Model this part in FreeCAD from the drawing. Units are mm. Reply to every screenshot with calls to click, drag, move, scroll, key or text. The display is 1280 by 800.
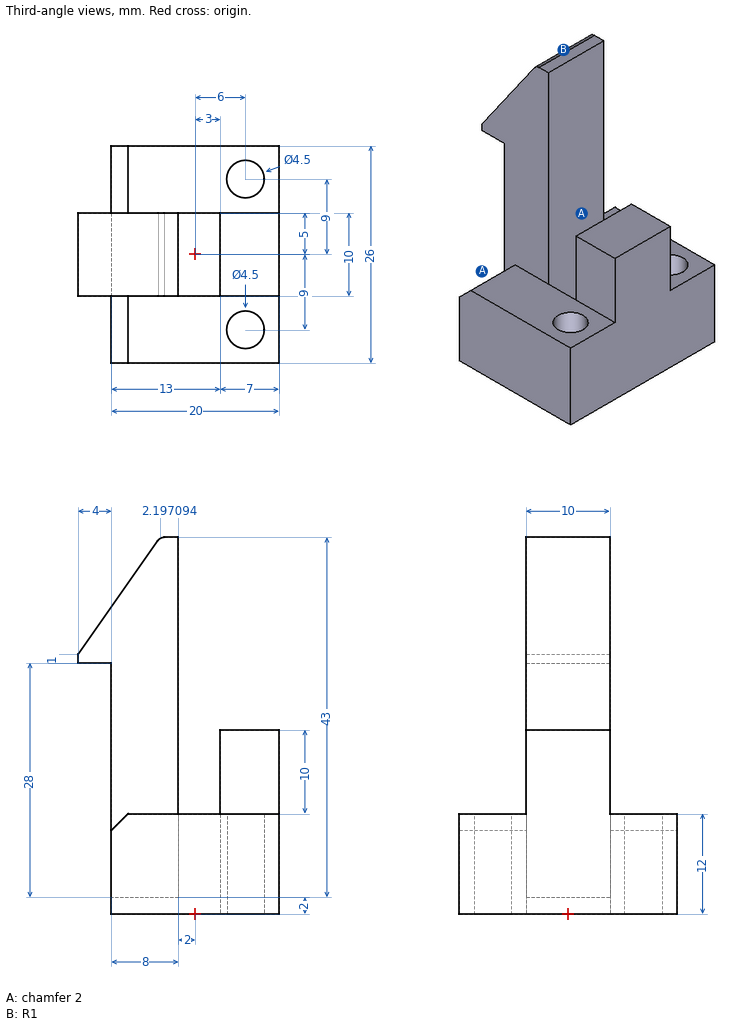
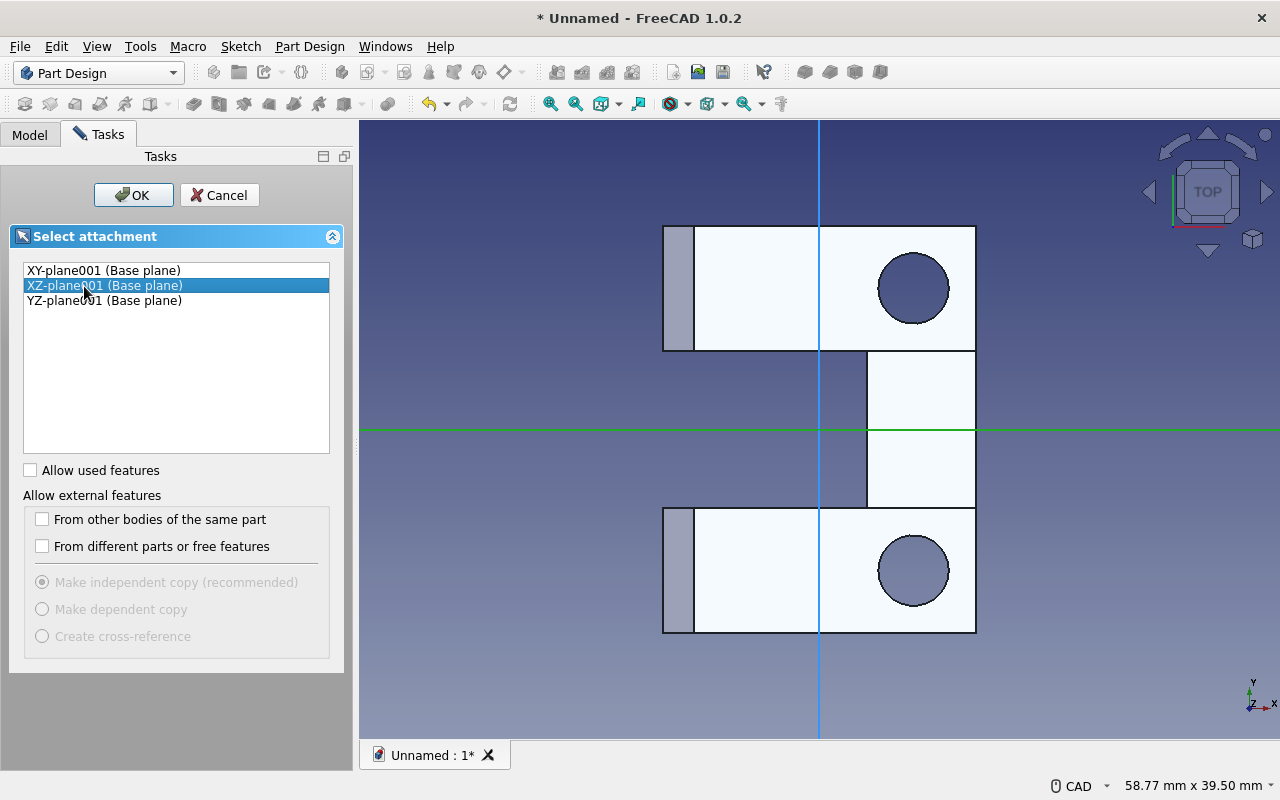
click(134, 195)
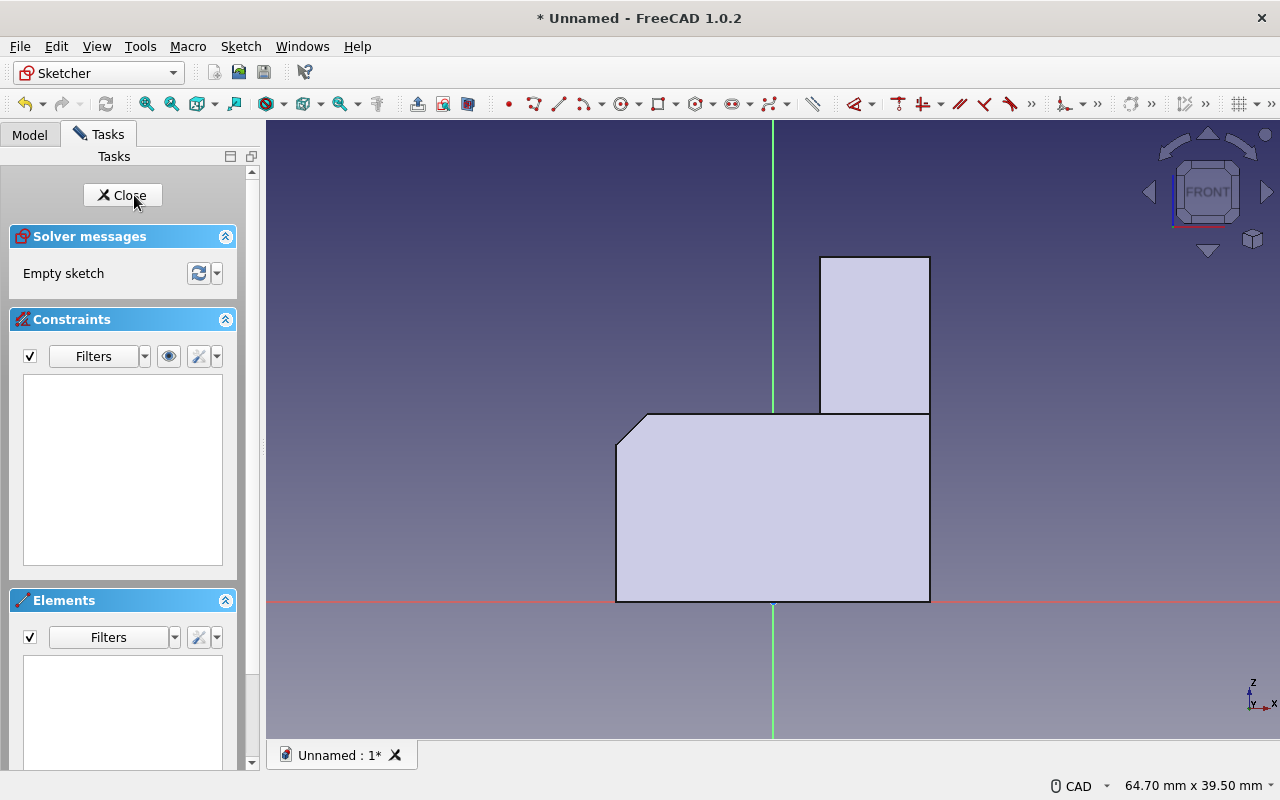
scroll(755, 649, down, 3)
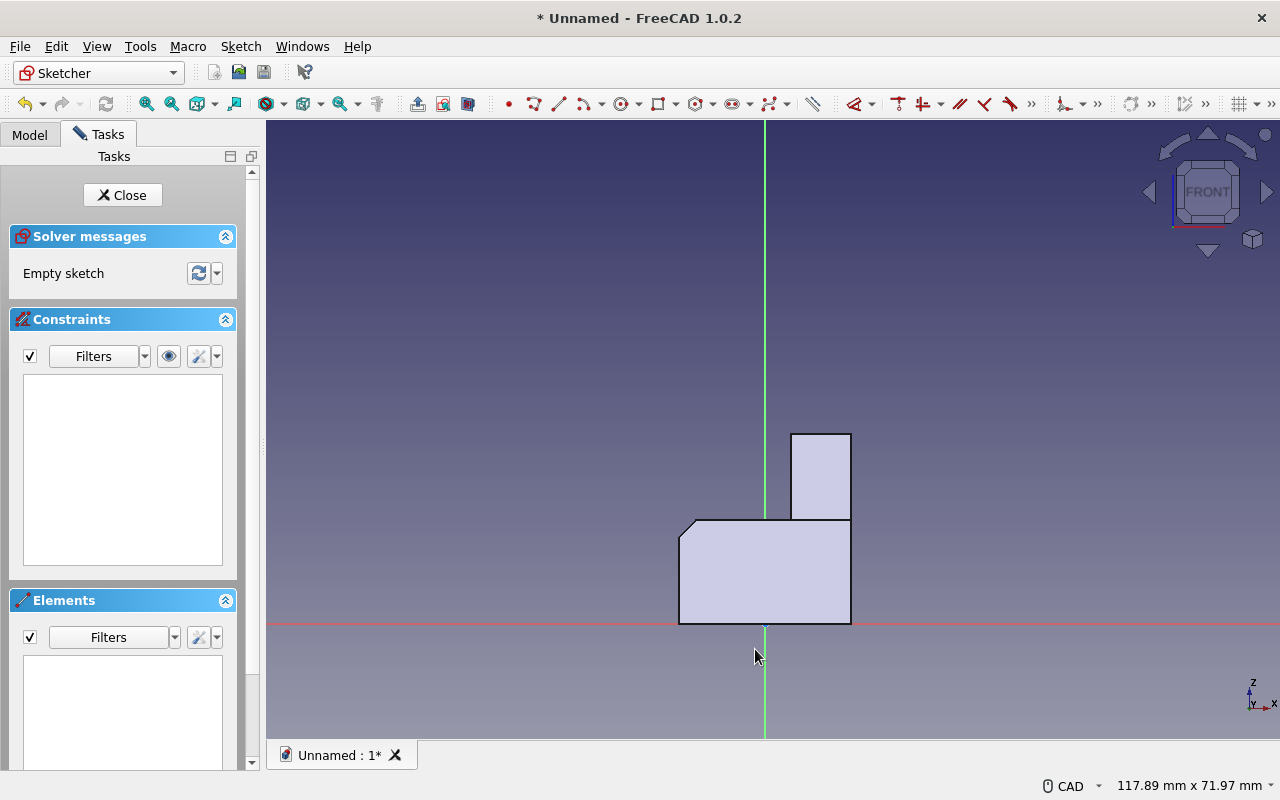
key(g)
key(m)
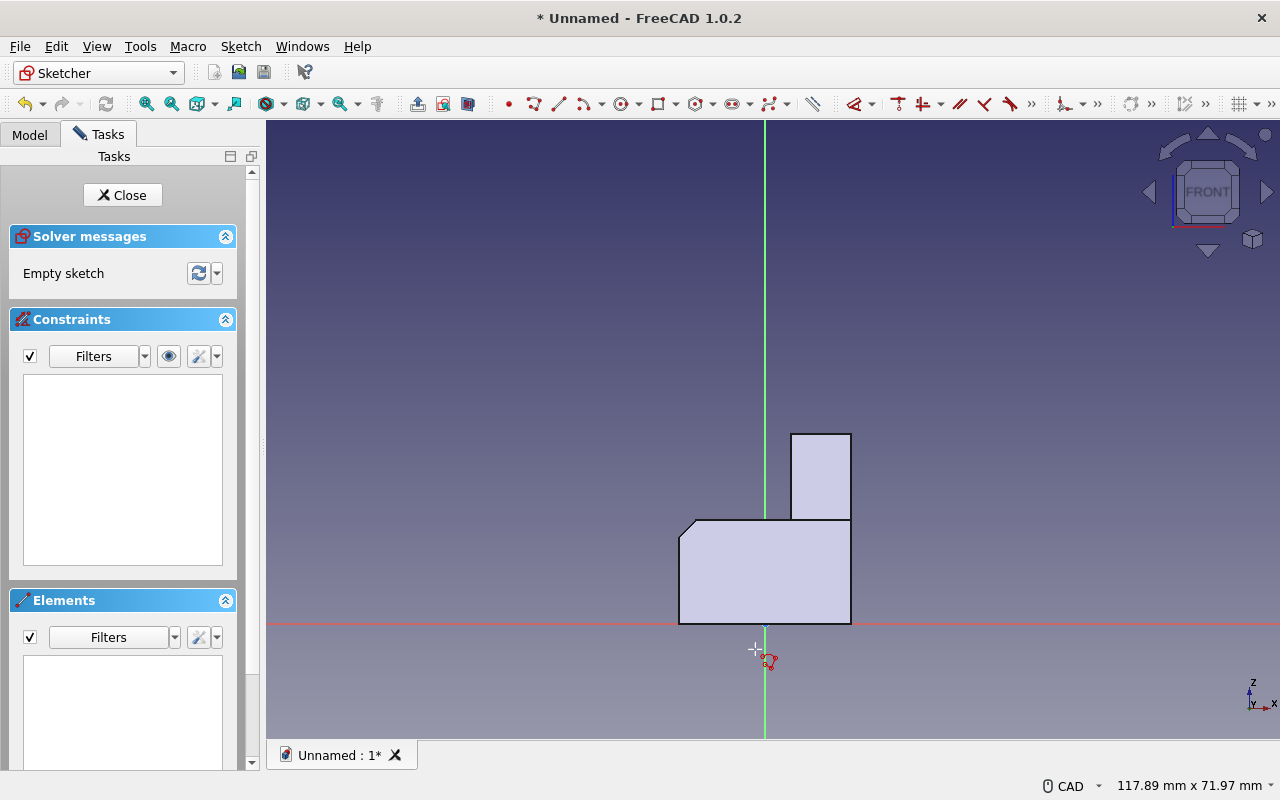
click(748, 606)
click(679, 606)
click(679, 366)
click(645, 366)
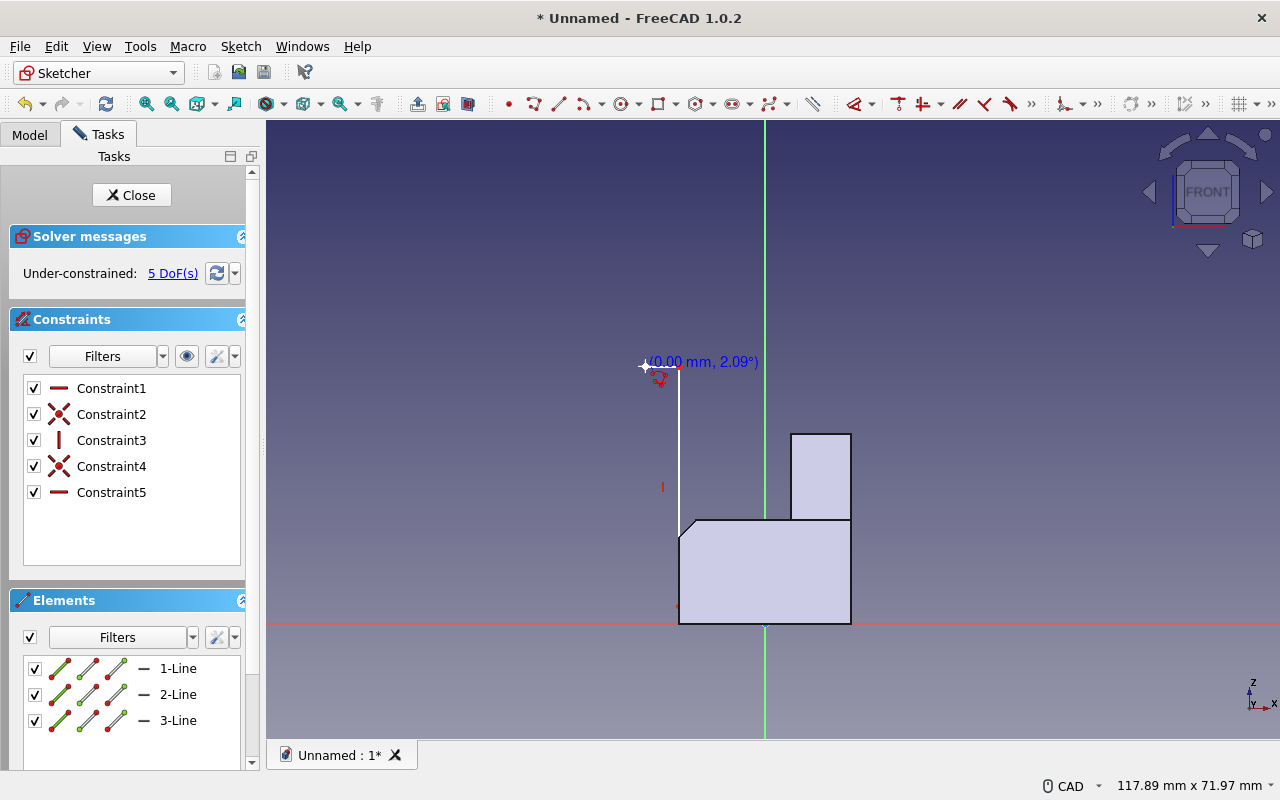
scroll(645, 357, up, 4)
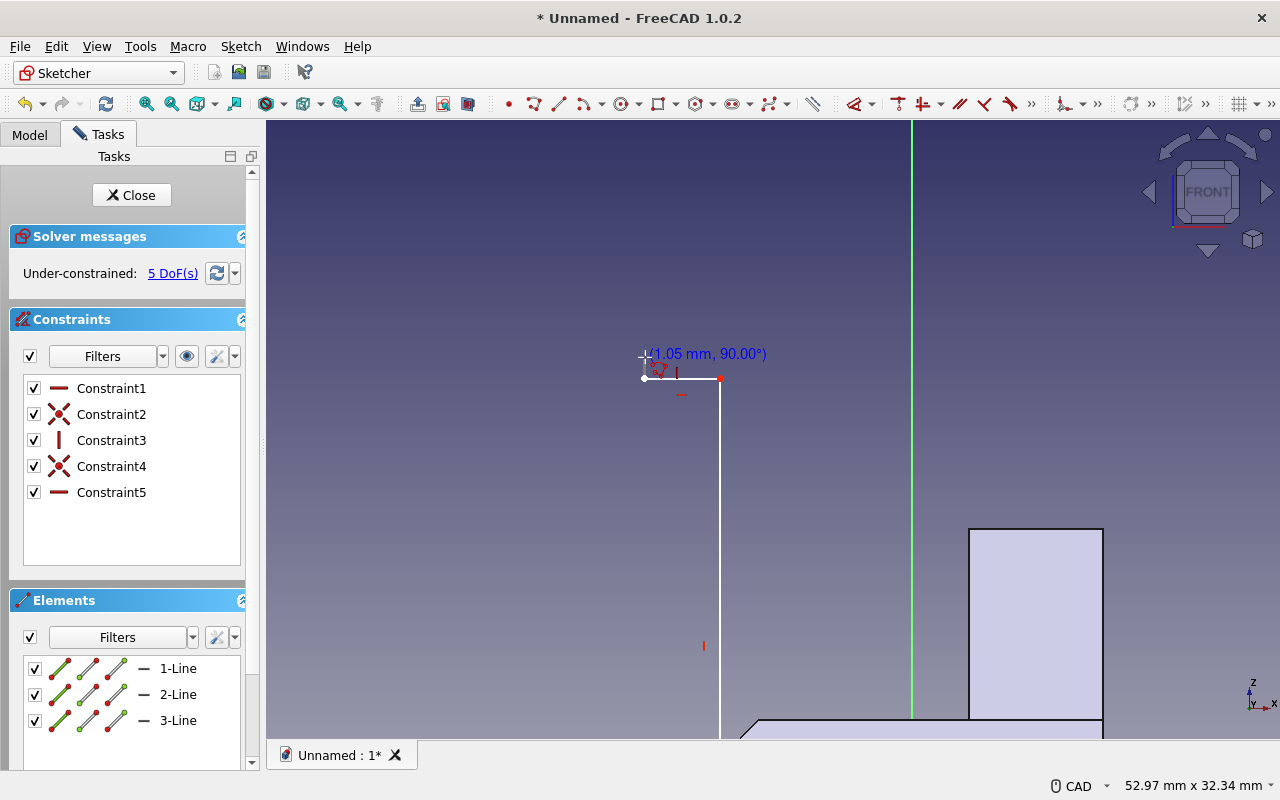
click(645, 356)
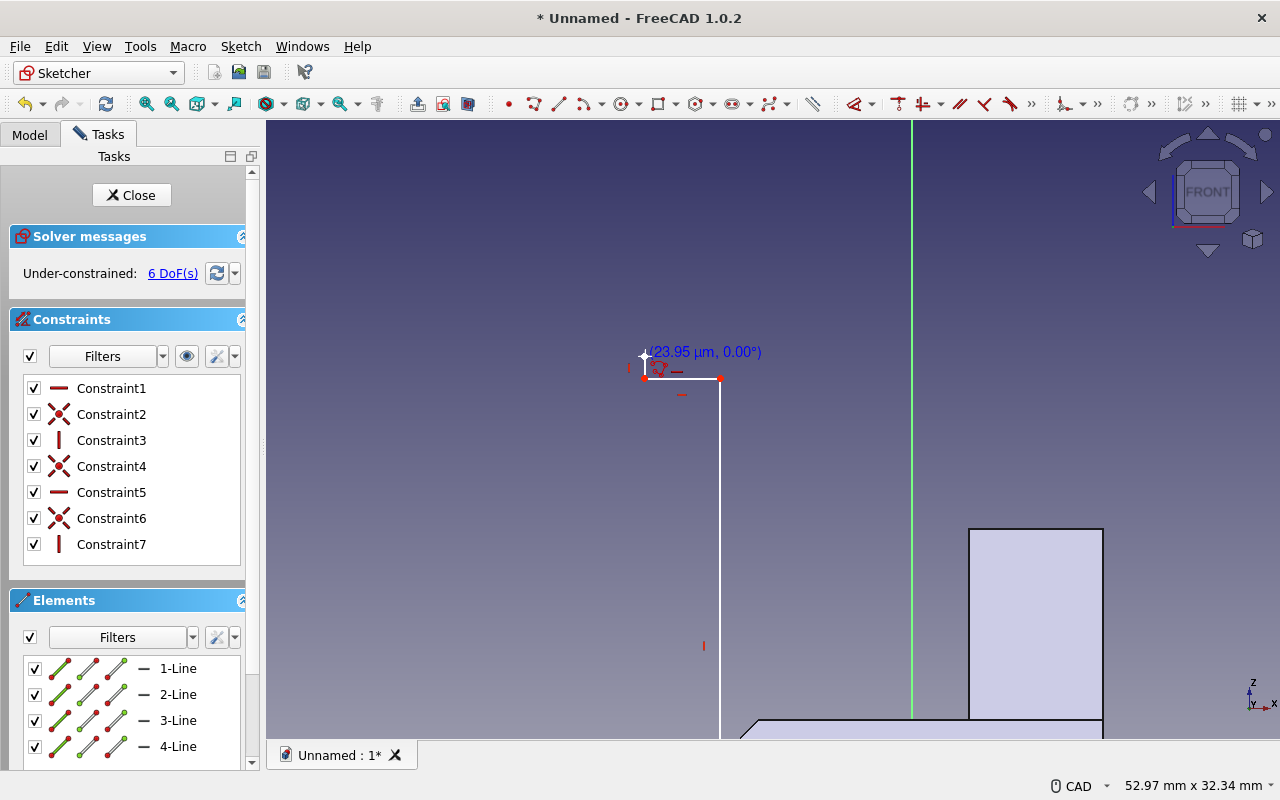
scroll(645, 356, down, 4)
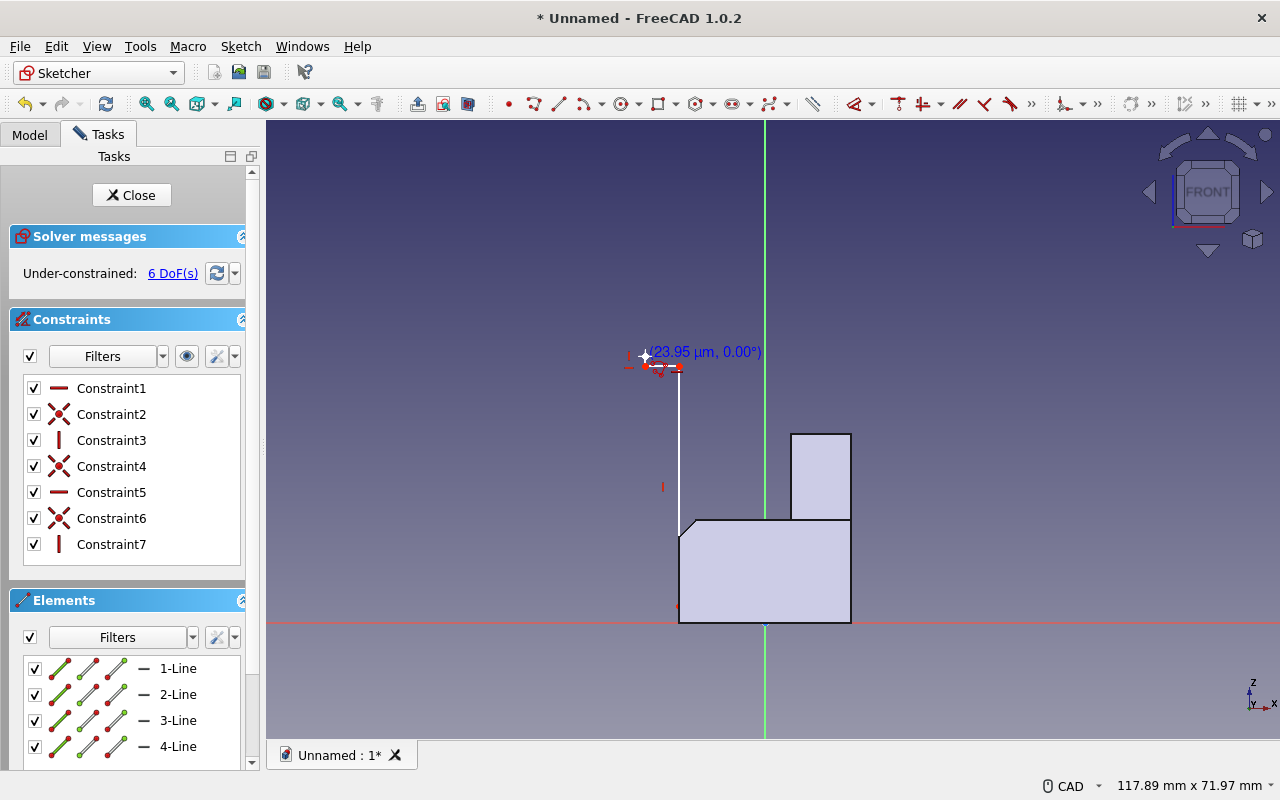
click(729, 236)
click(748, 236)
click(748, 606)
key(Escape)
key(Escape)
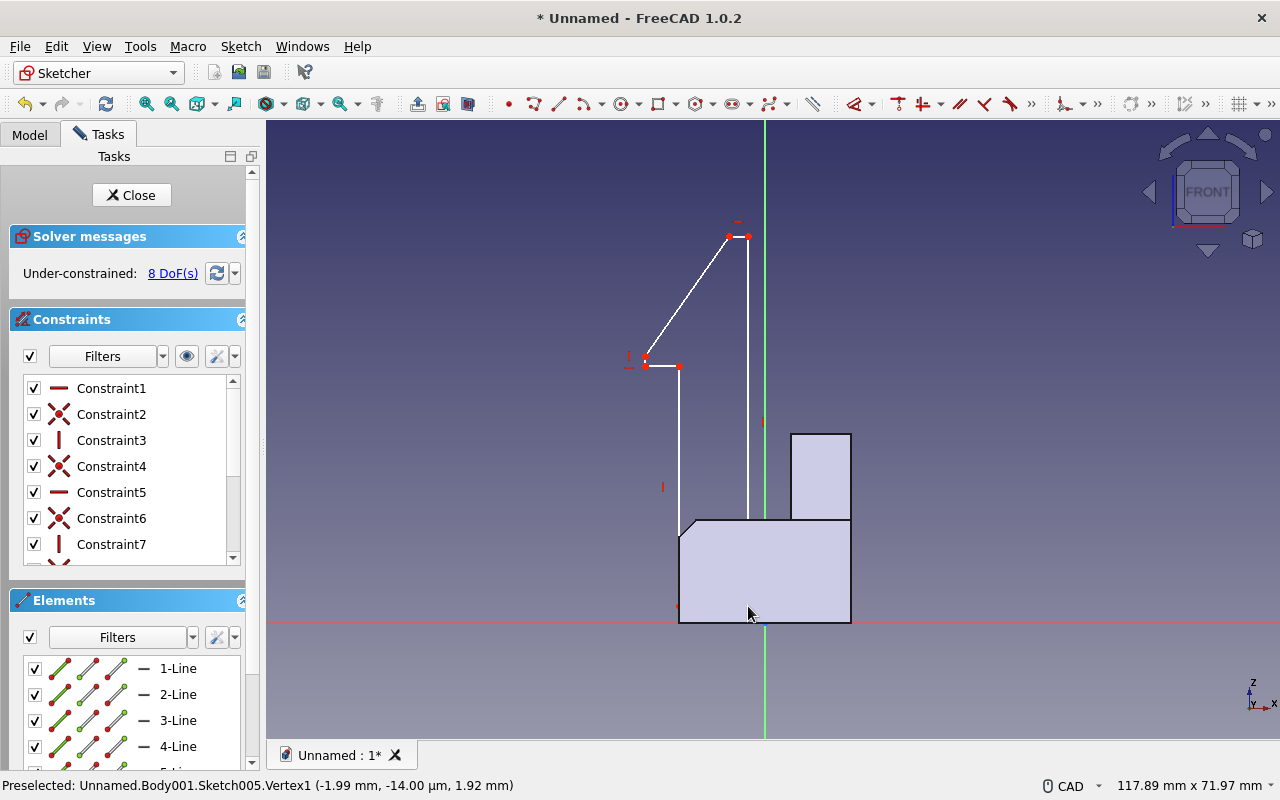
click(854, 104)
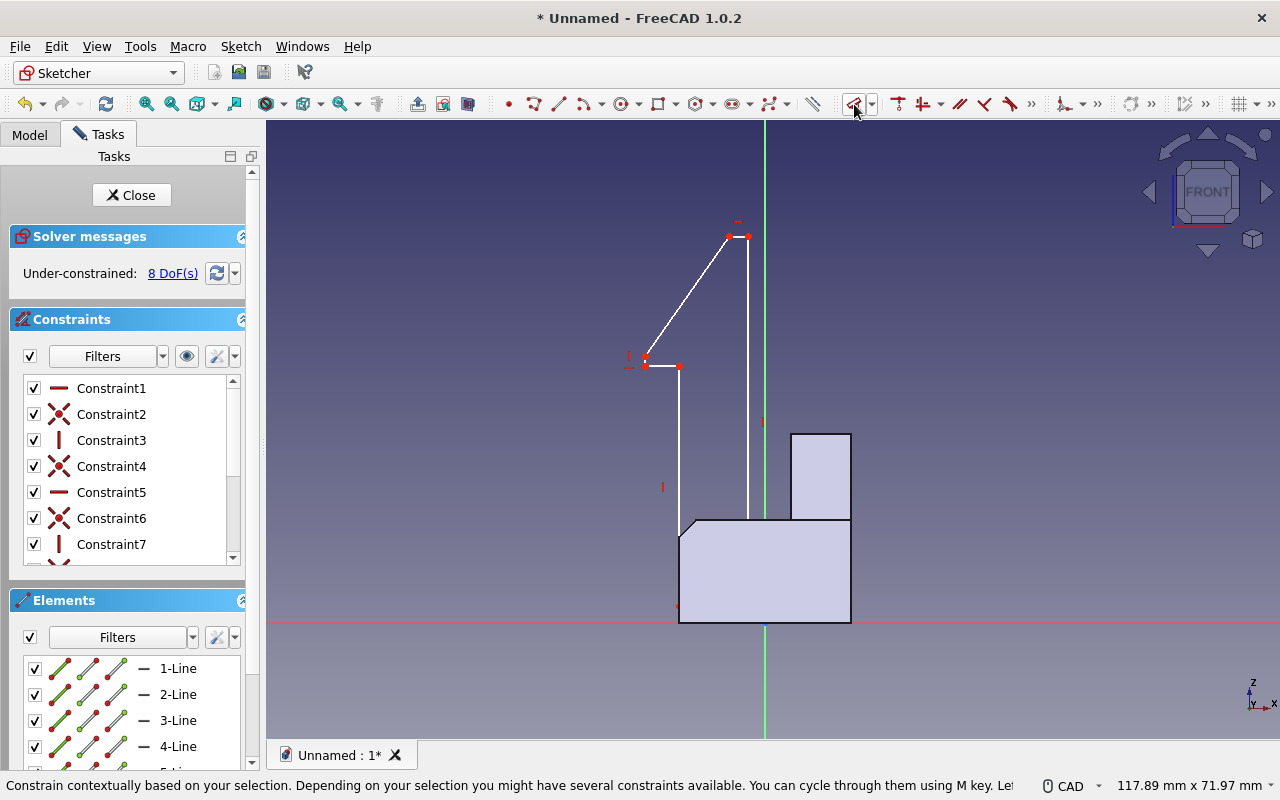
click(727, 606)
click(713, 640)